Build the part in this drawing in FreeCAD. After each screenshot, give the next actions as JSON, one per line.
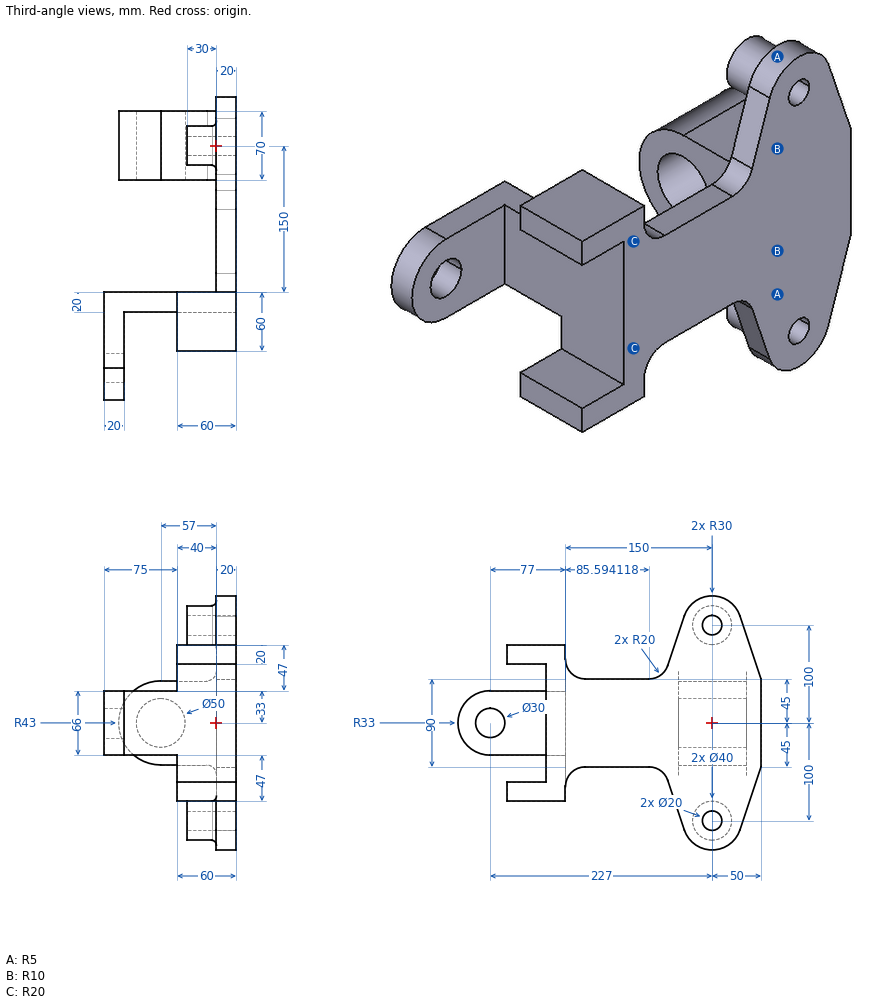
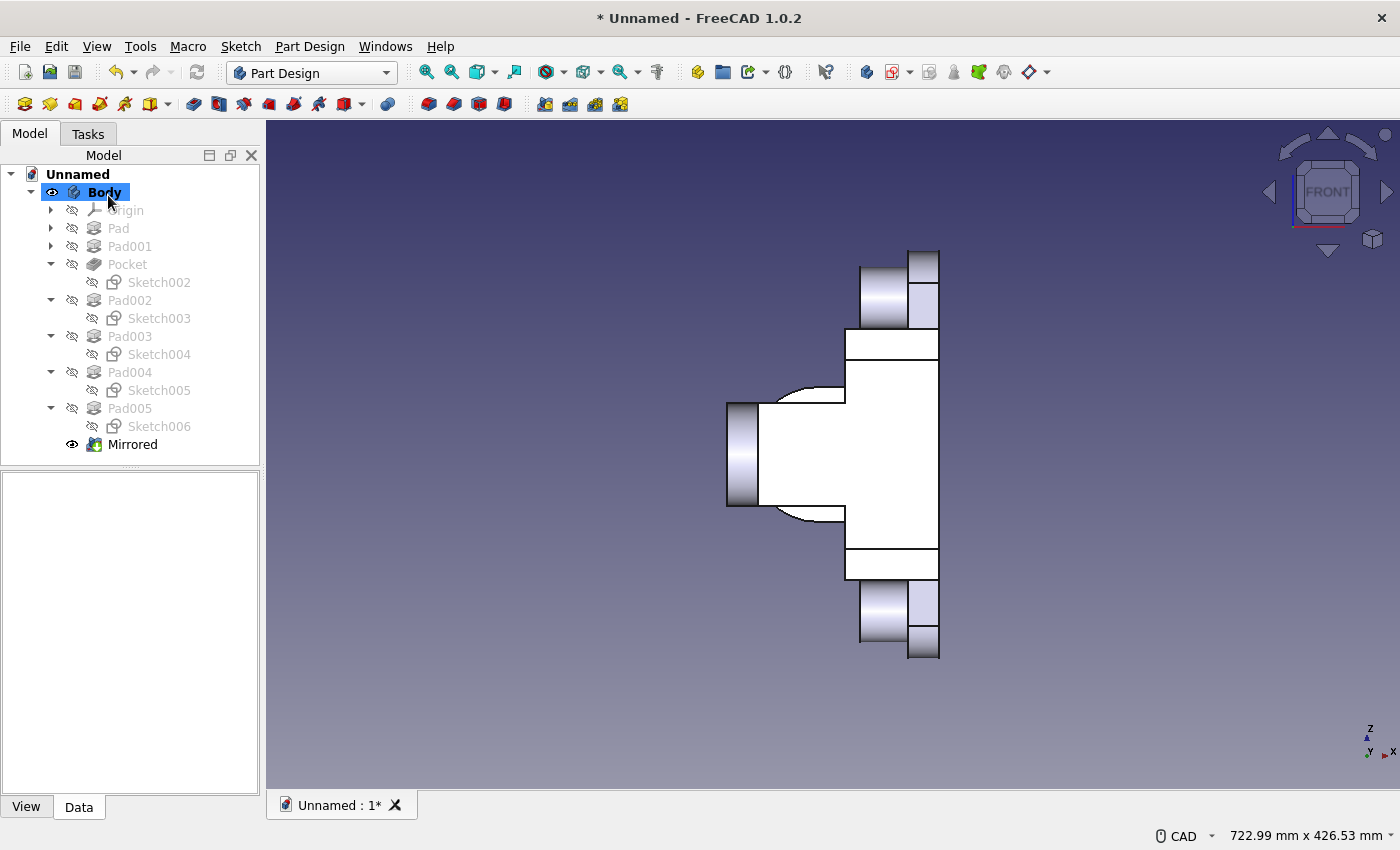
{"action": "key", "text": "3"}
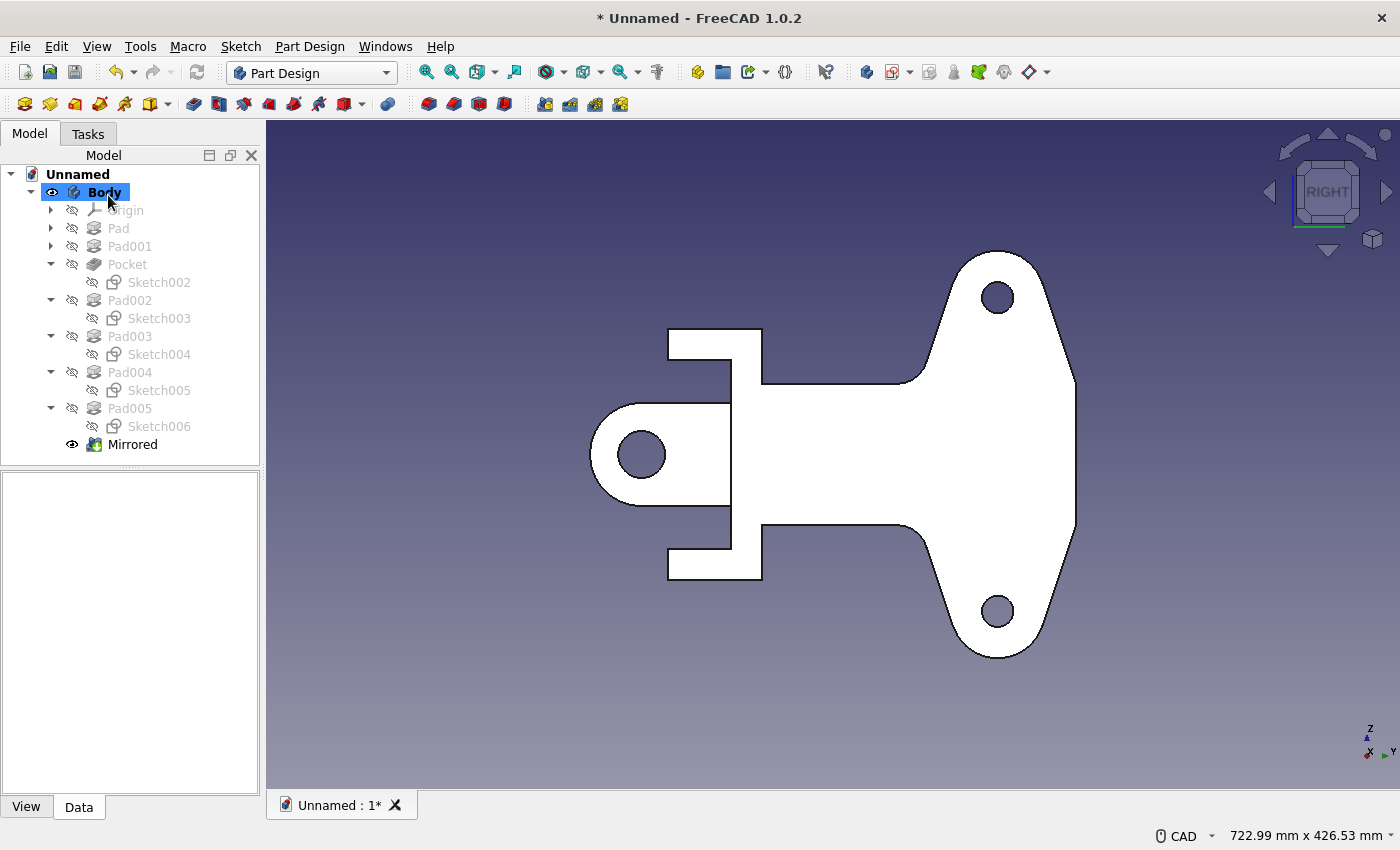
{"action": "key", "text": "5"}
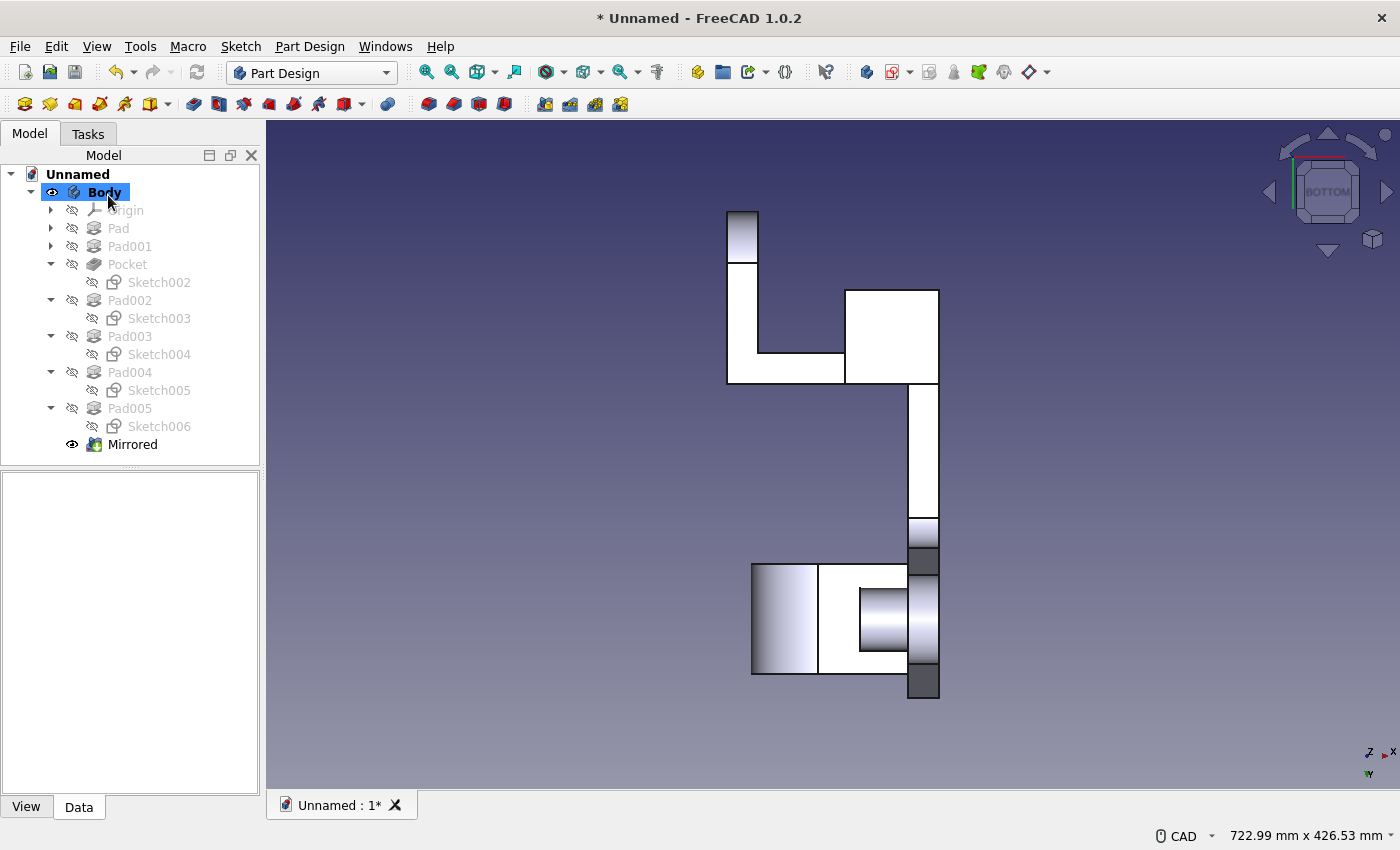
{"action": "key", "text": "4"}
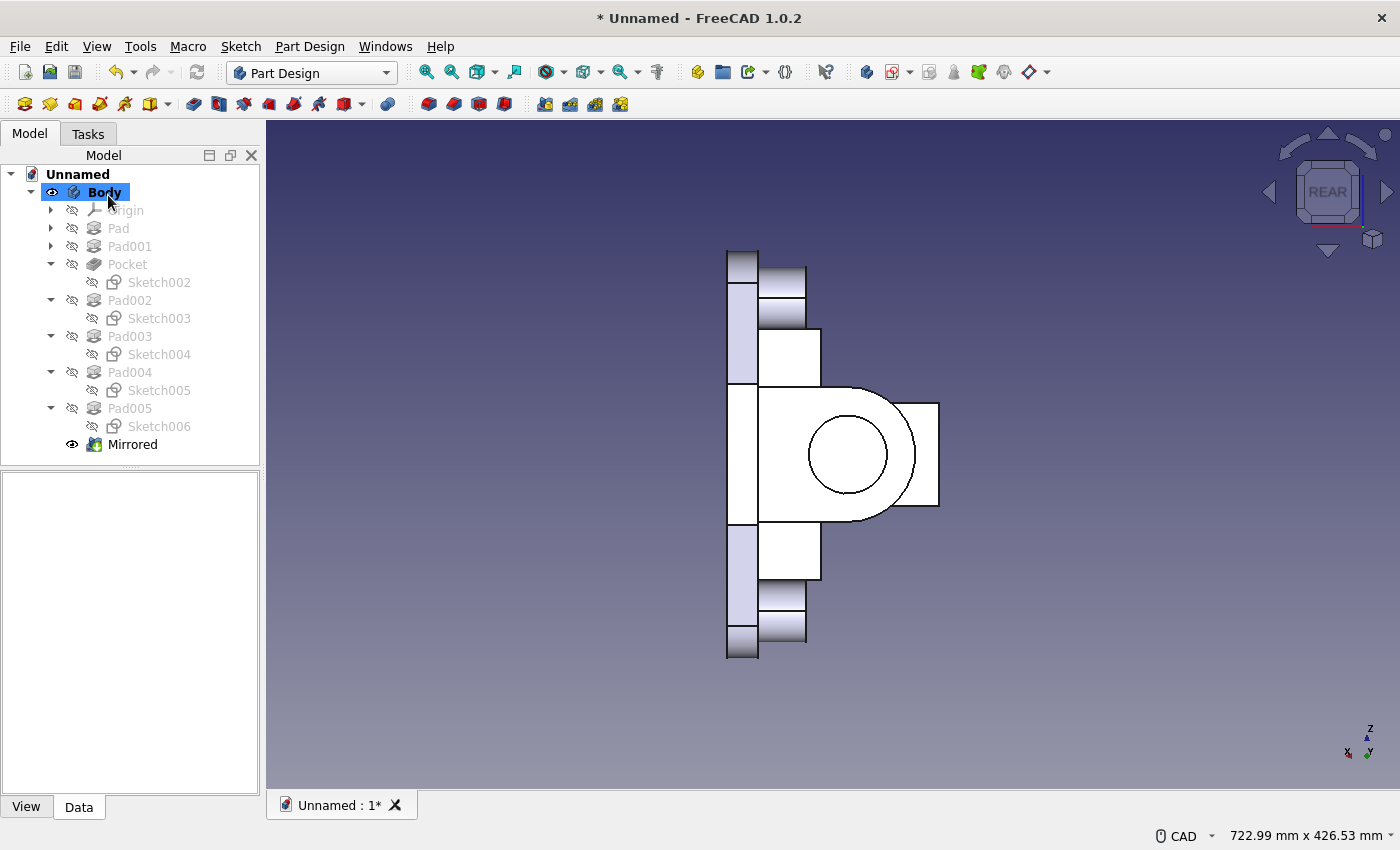
{"action": "key", "text": "6"}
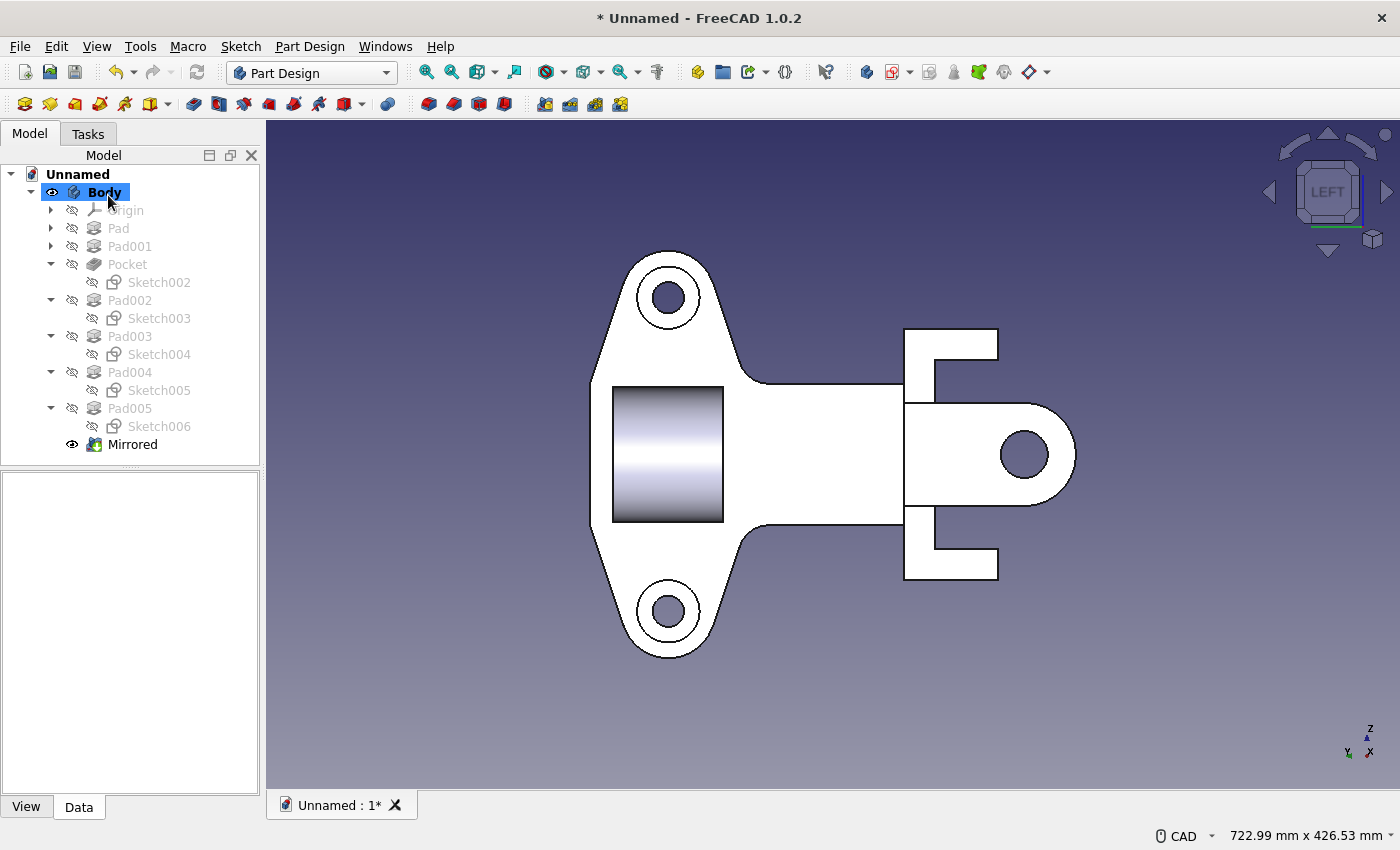
{"action": "key", "text": "v 3"}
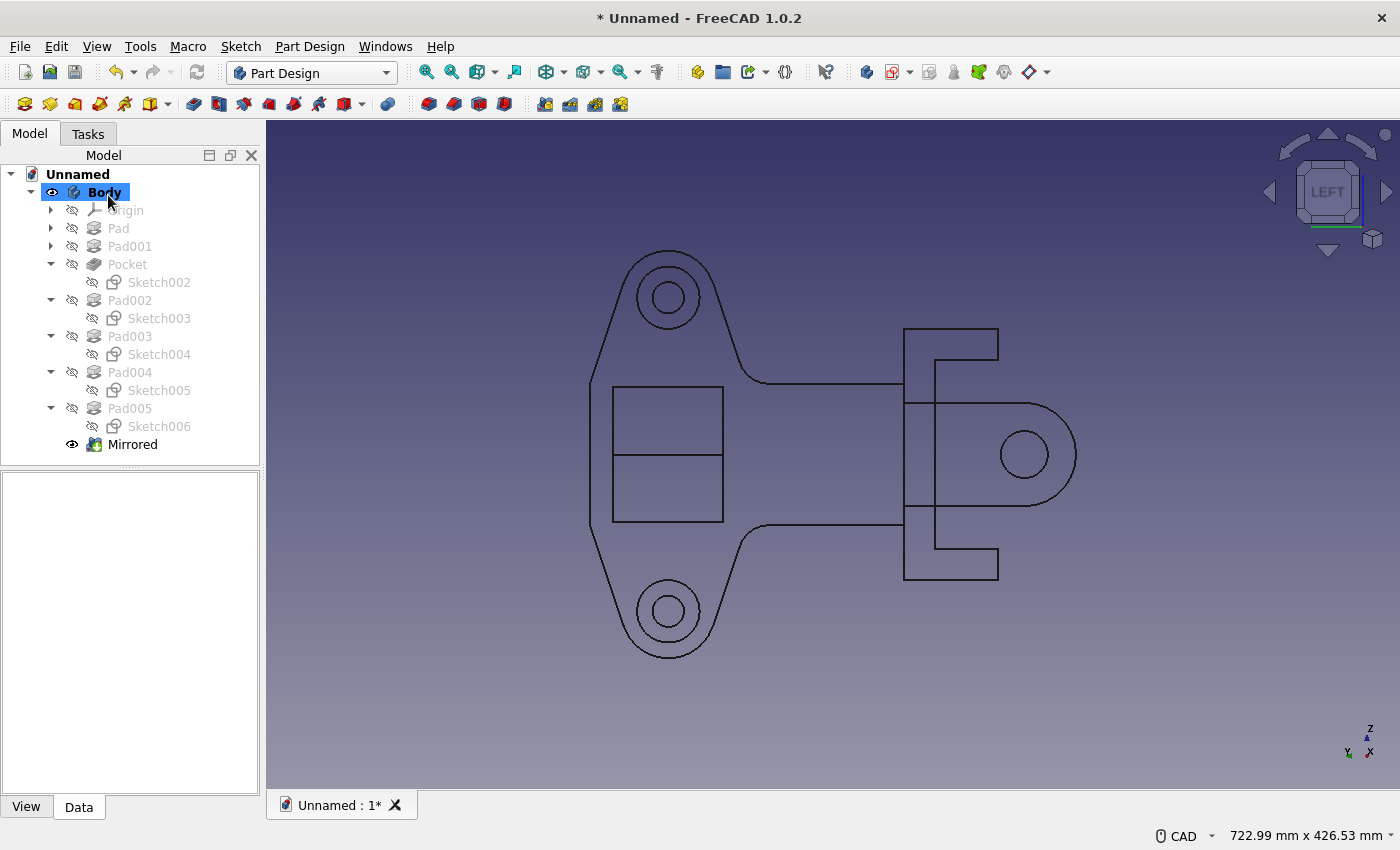
{"action": "key", "text": "0"}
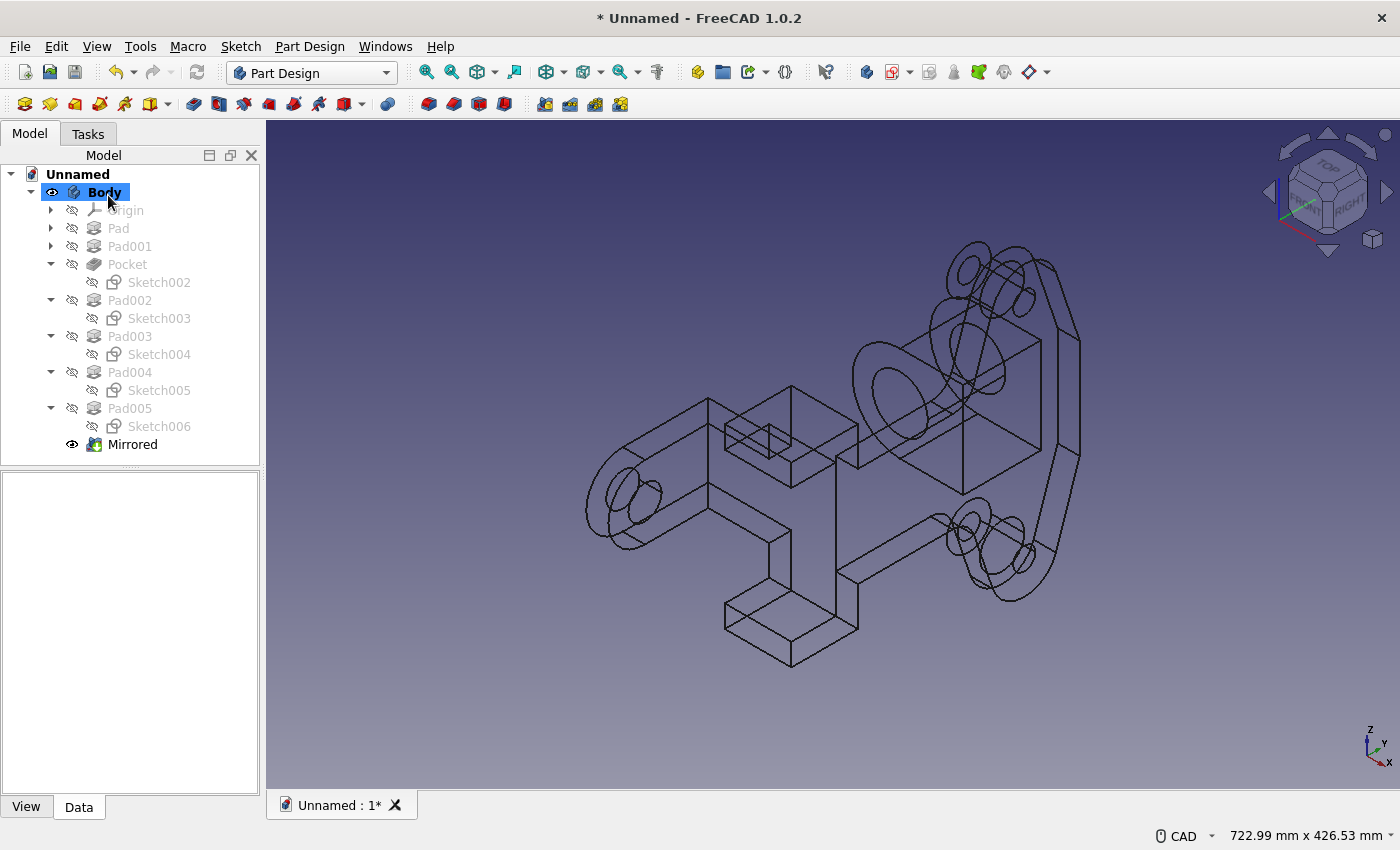
{"action": "left_click", "coordinate": [984, 540]}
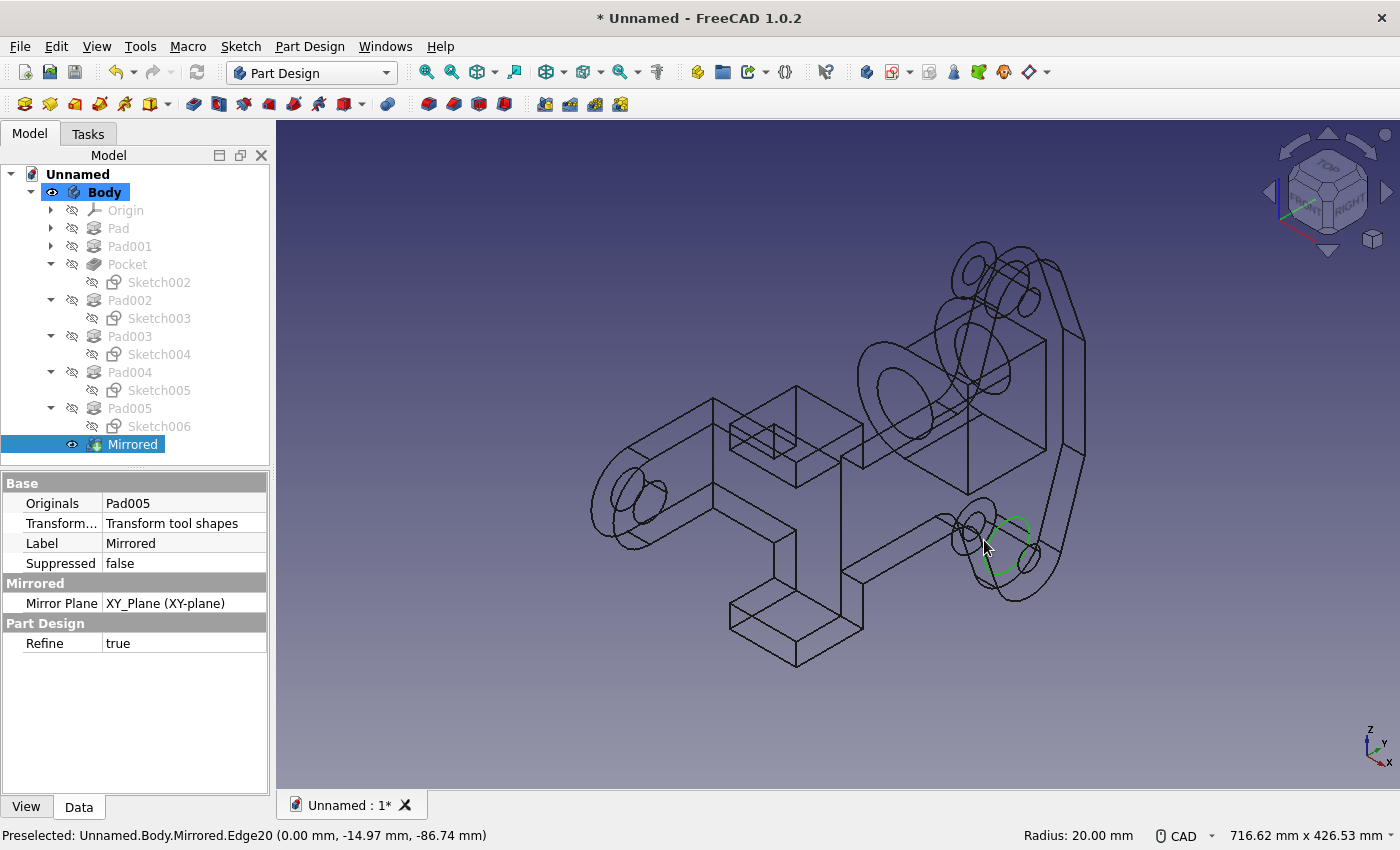
{"action": "left_click", "coordinate": [989, 284], "text": "ctrl"}